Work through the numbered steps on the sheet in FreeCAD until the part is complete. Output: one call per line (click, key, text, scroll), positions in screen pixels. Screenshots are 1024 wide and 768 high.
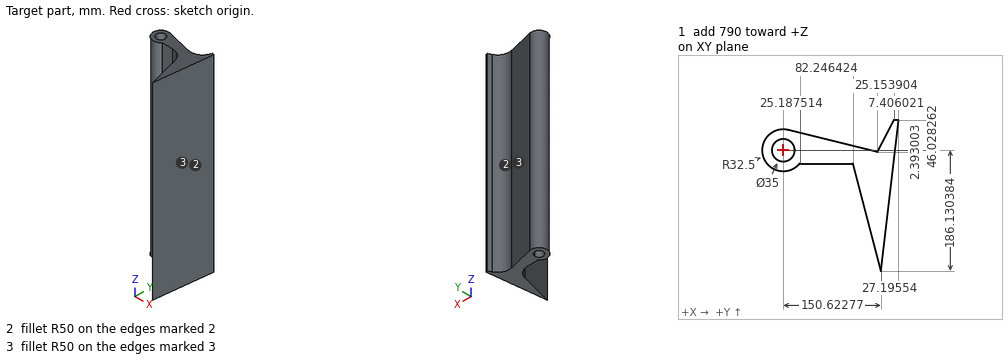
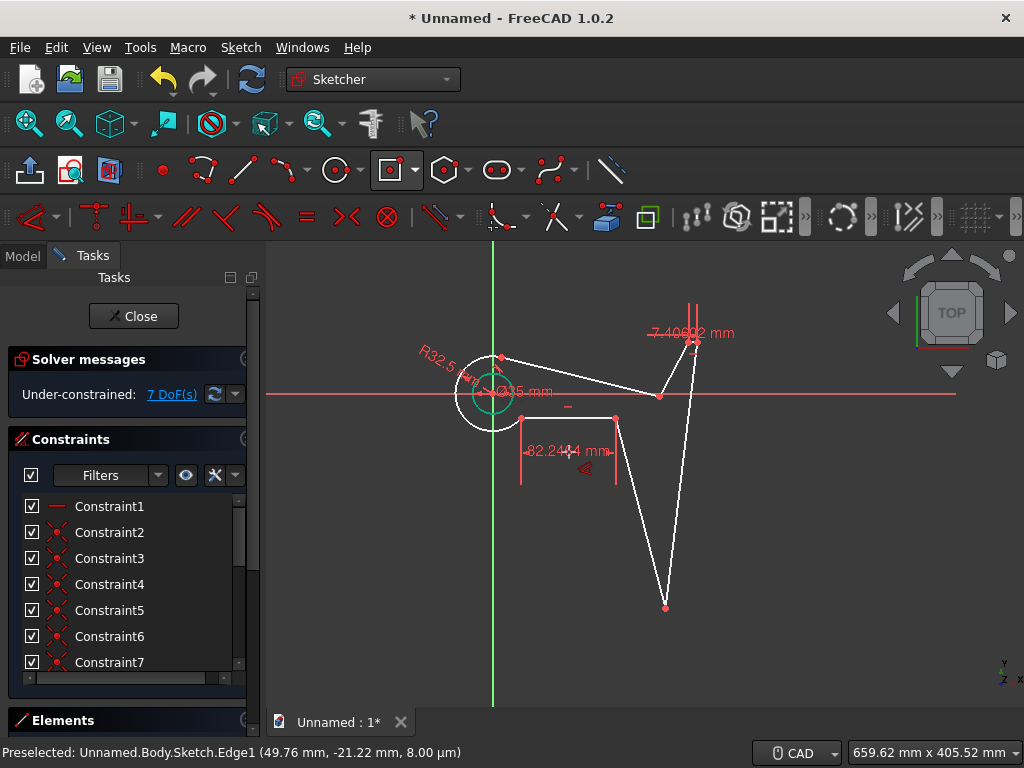
scroll(660, 397, up, 14)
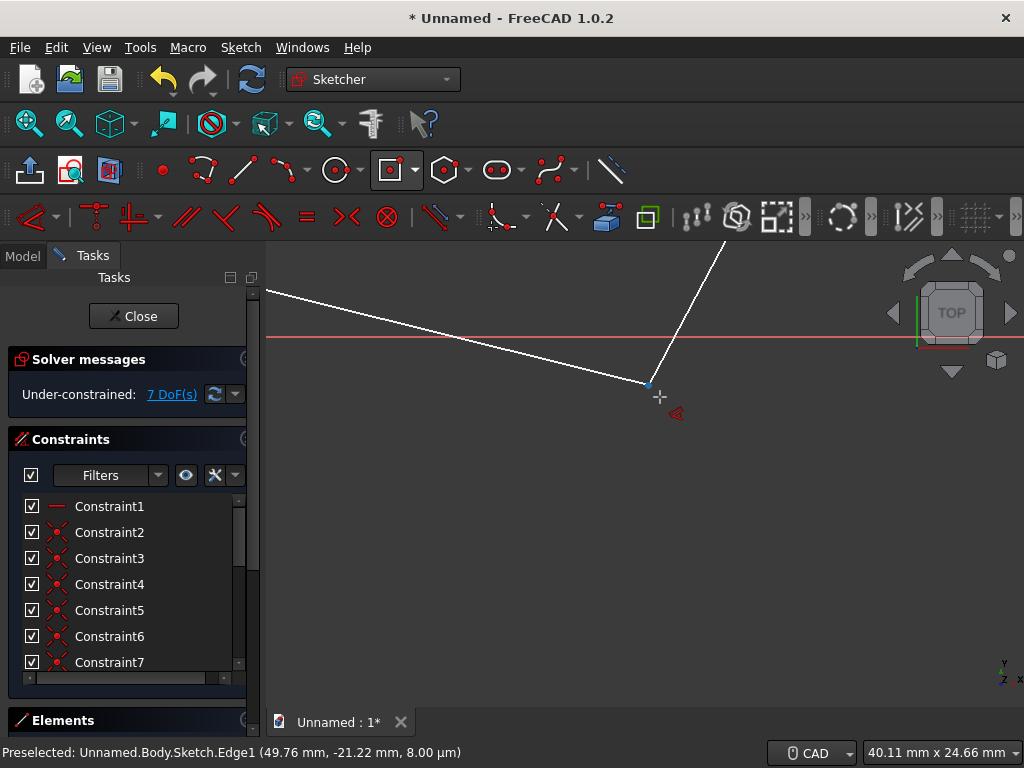
click(649, 385)
click(683, 361)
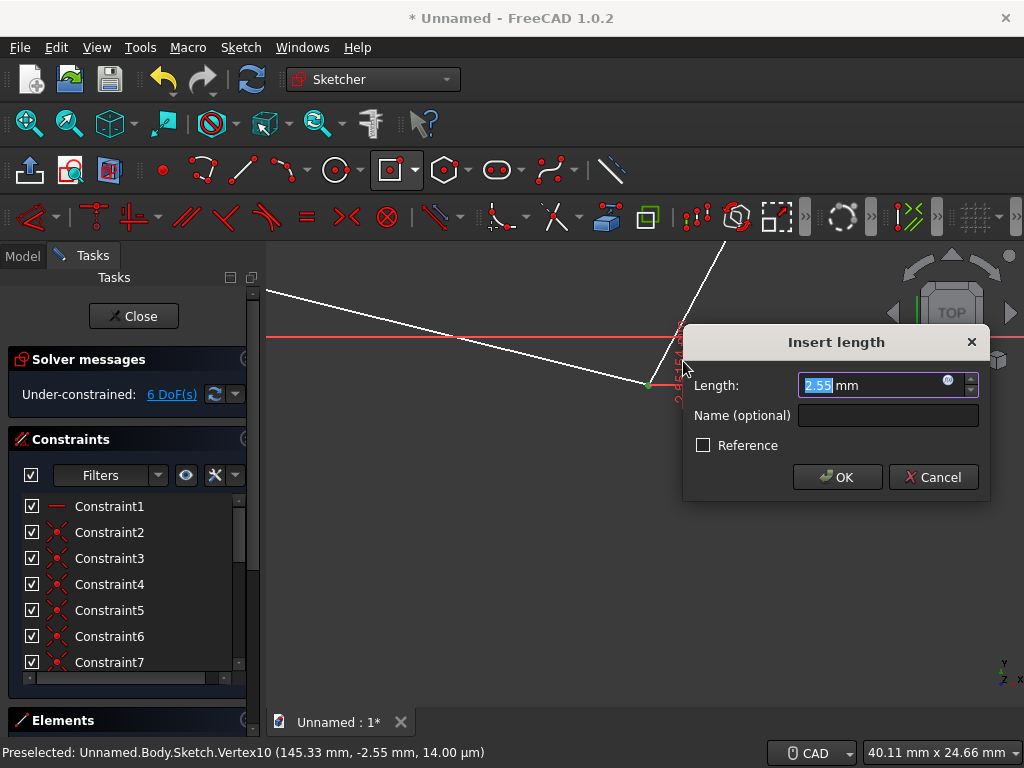
text(2.393003)
key(Return)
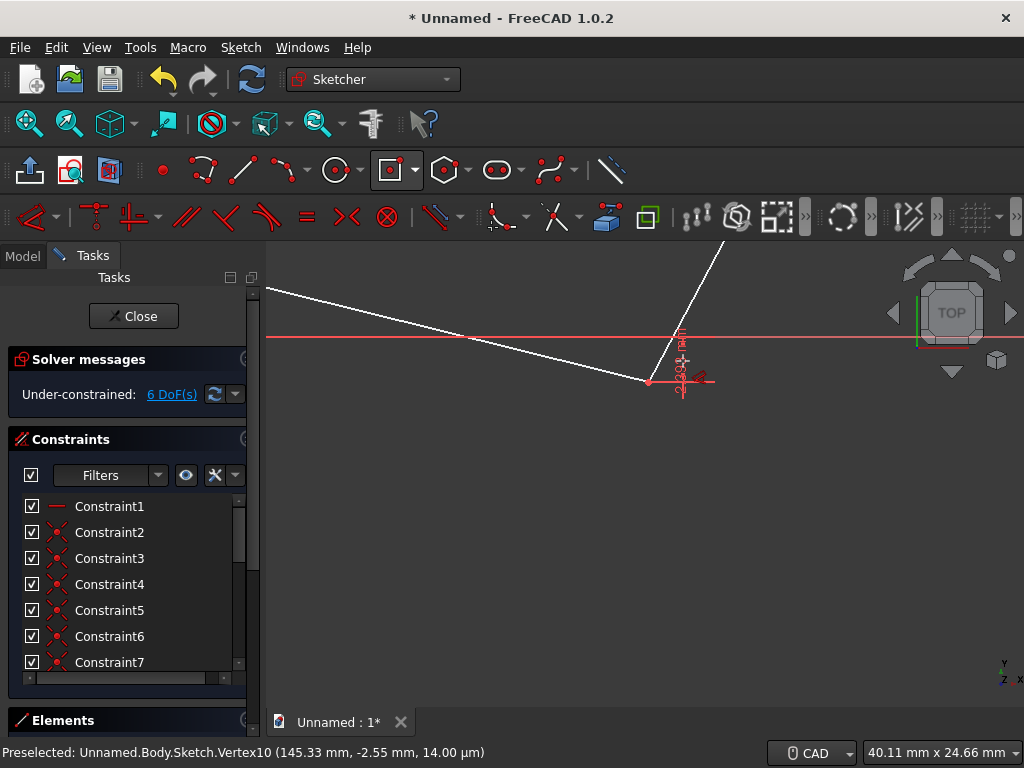
scroll(660, 397, down, 14)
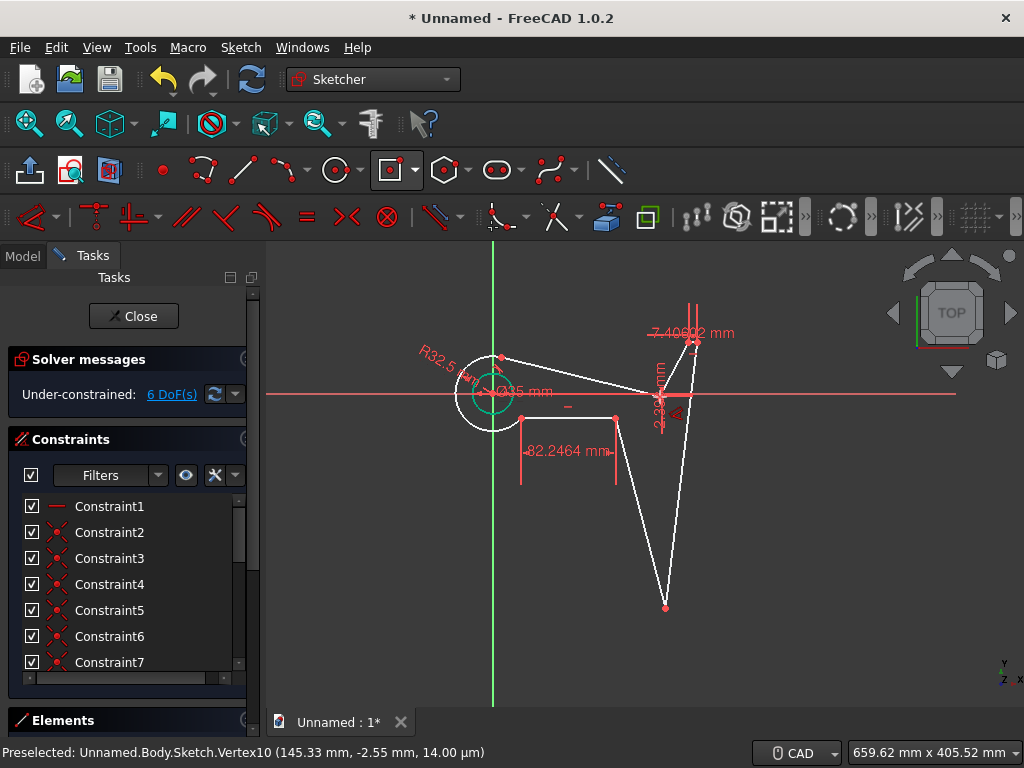
scroll(675, 528, up, 2)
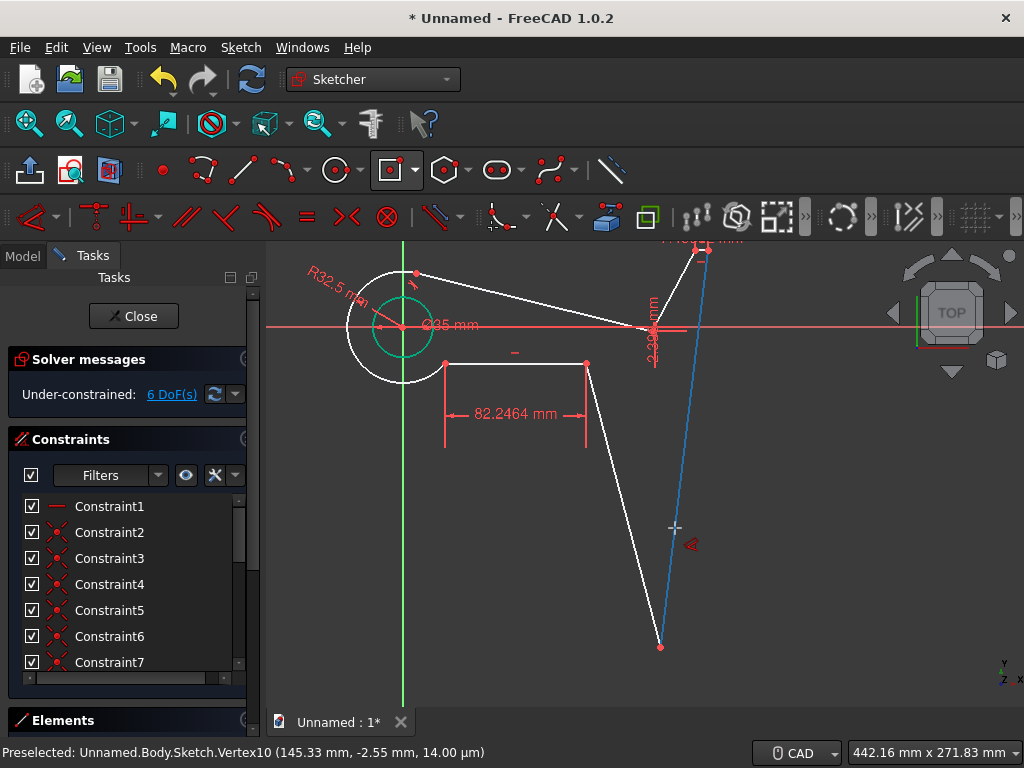
click(675, 528)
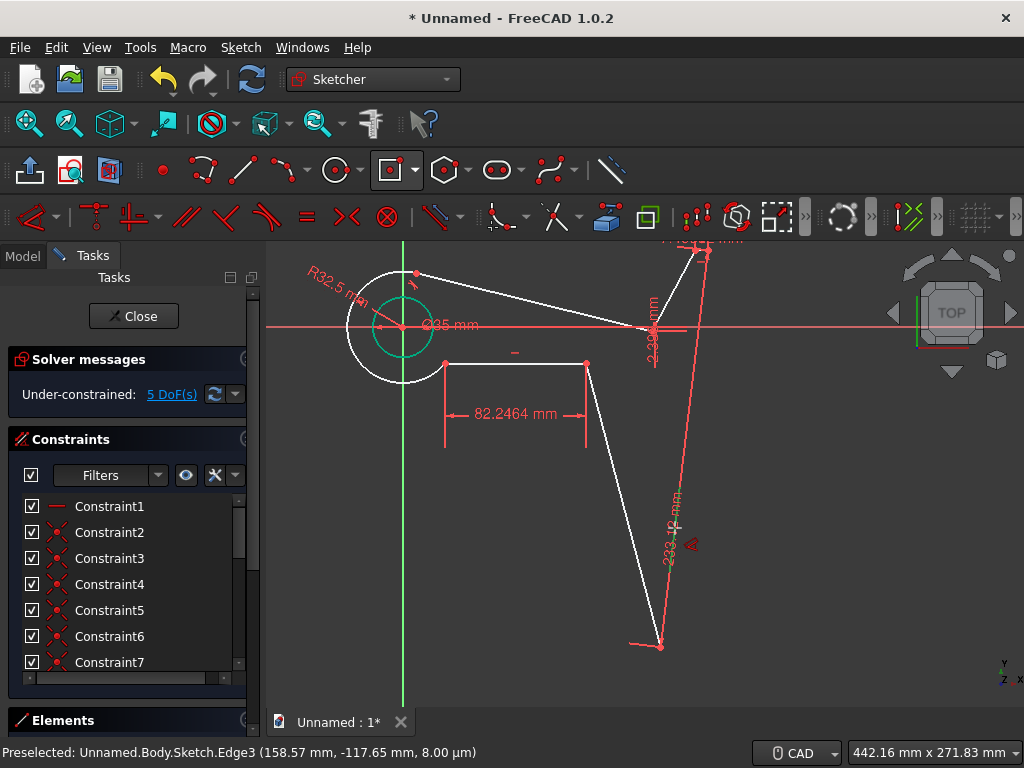
key(Escape)
key(Escape)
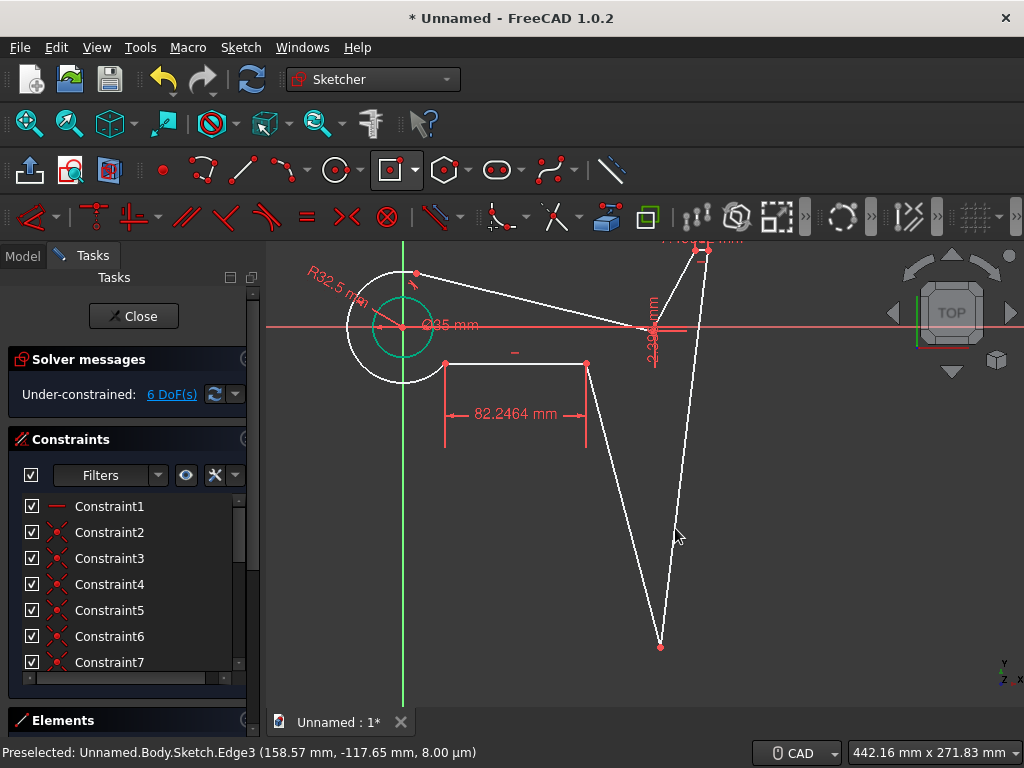
click(675, 528)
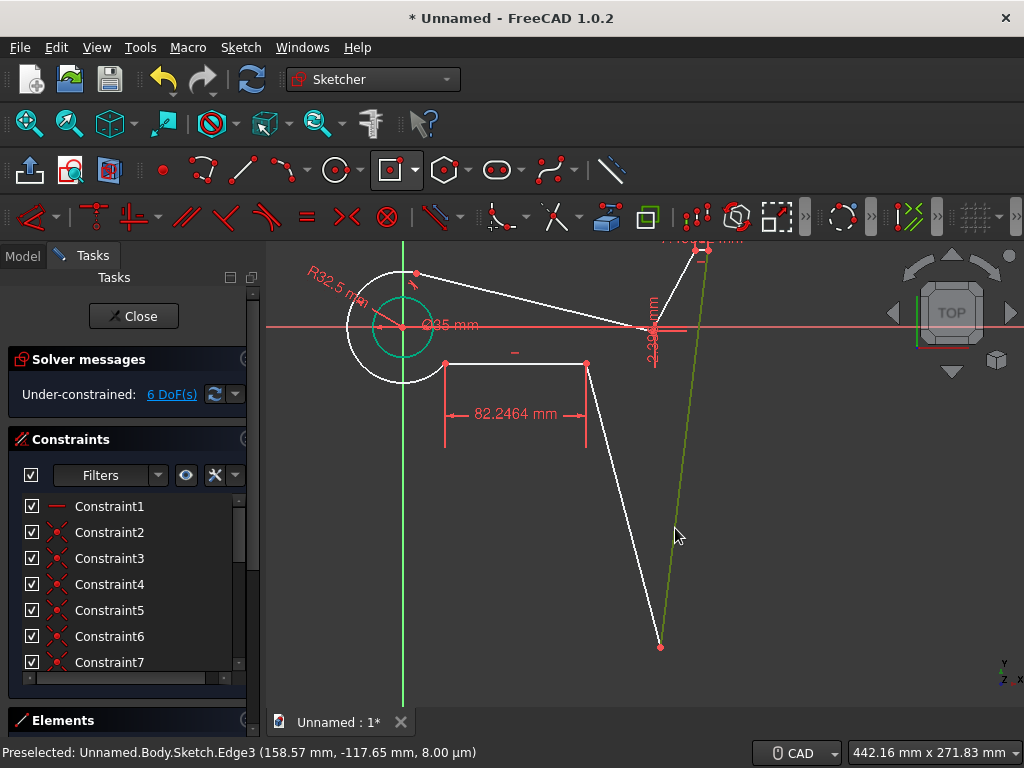
key(l)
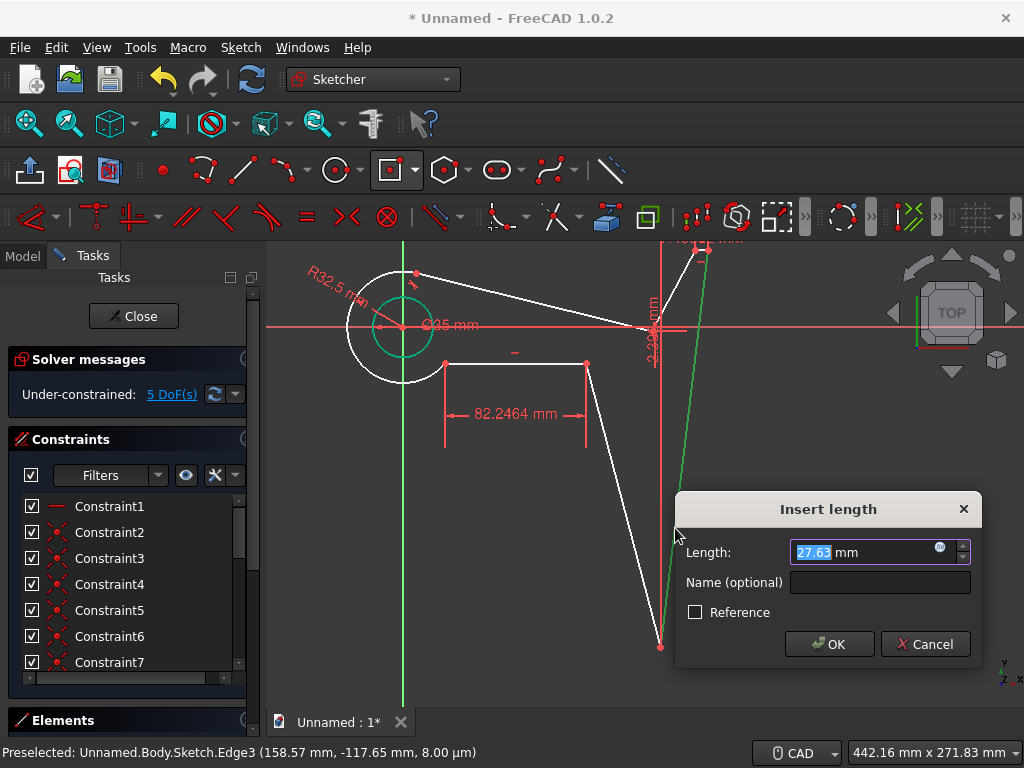
text(27.19554)
key(Return)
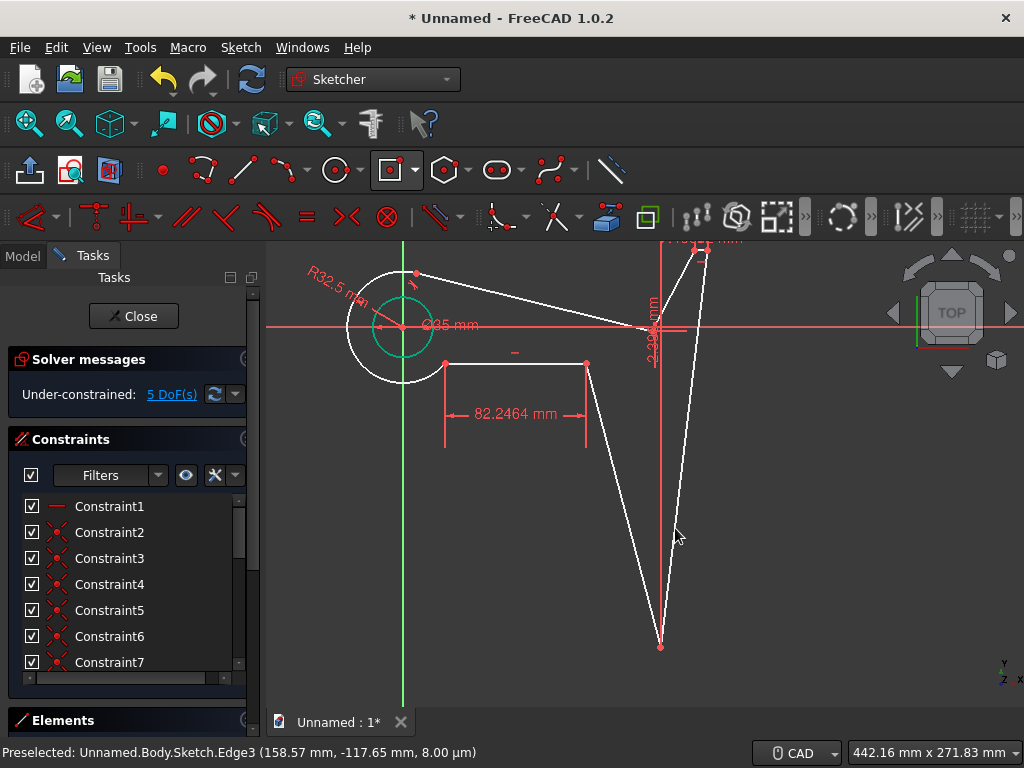
click(445, 364)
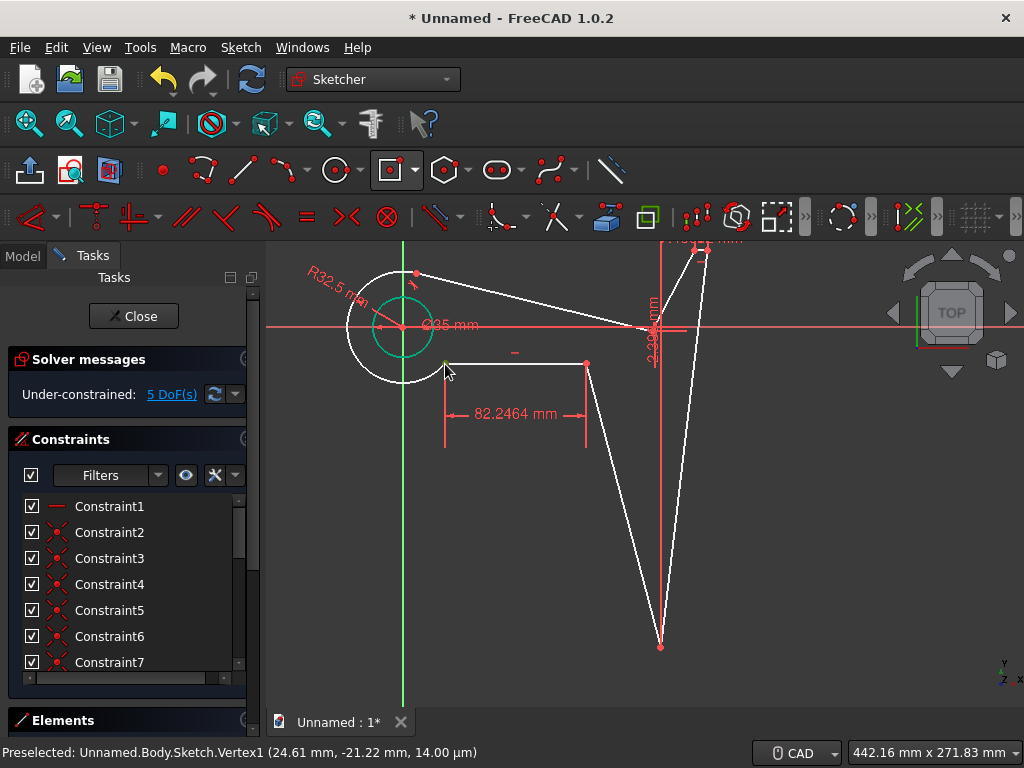
click(58, 218)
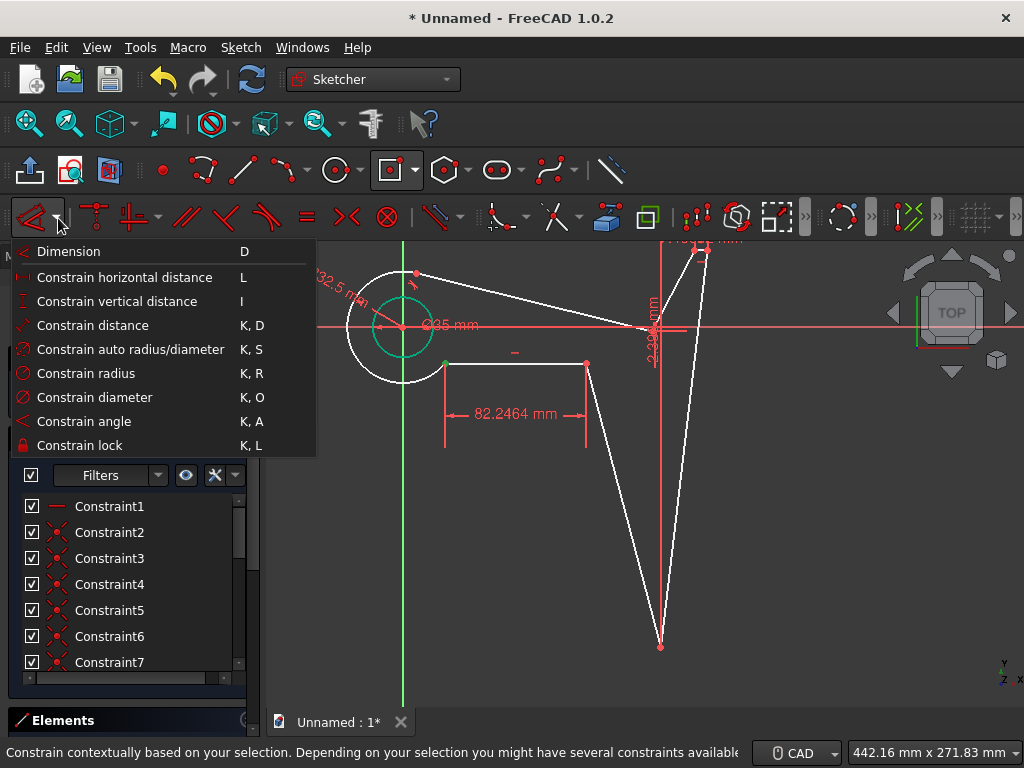
click(164, 277)